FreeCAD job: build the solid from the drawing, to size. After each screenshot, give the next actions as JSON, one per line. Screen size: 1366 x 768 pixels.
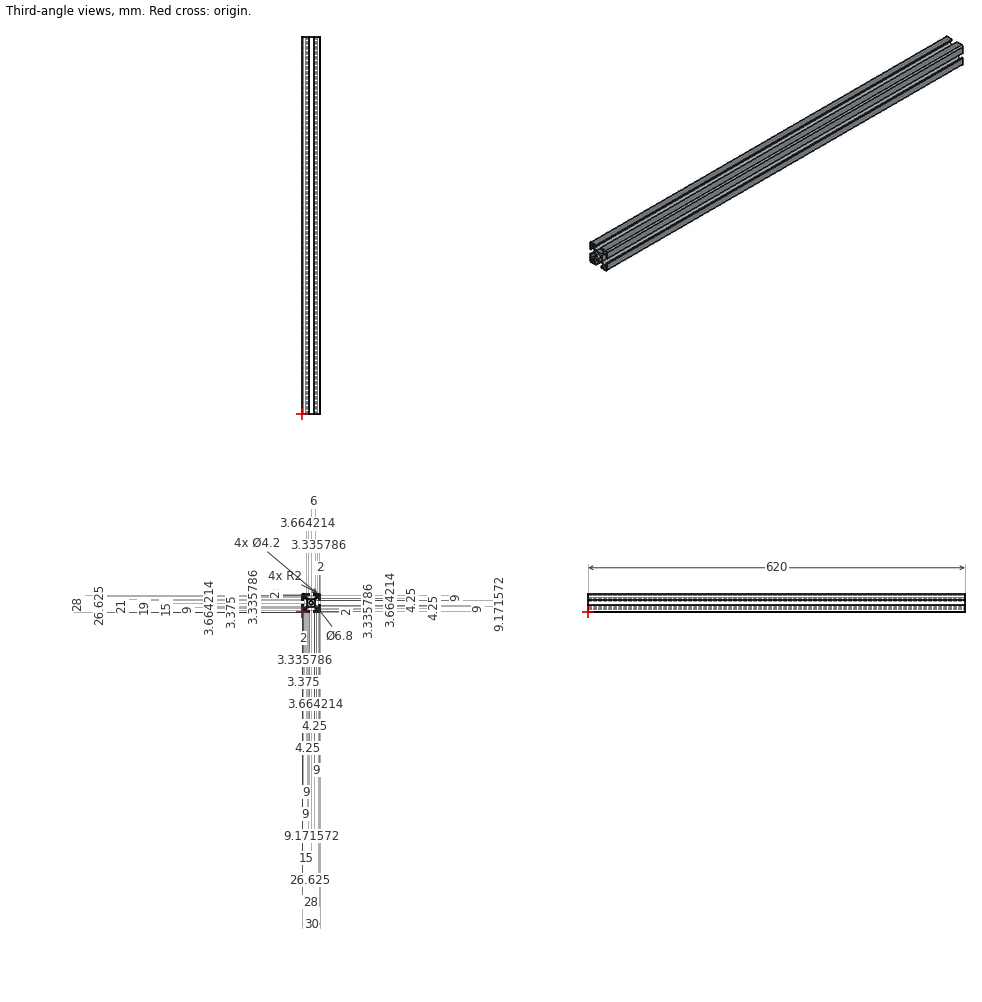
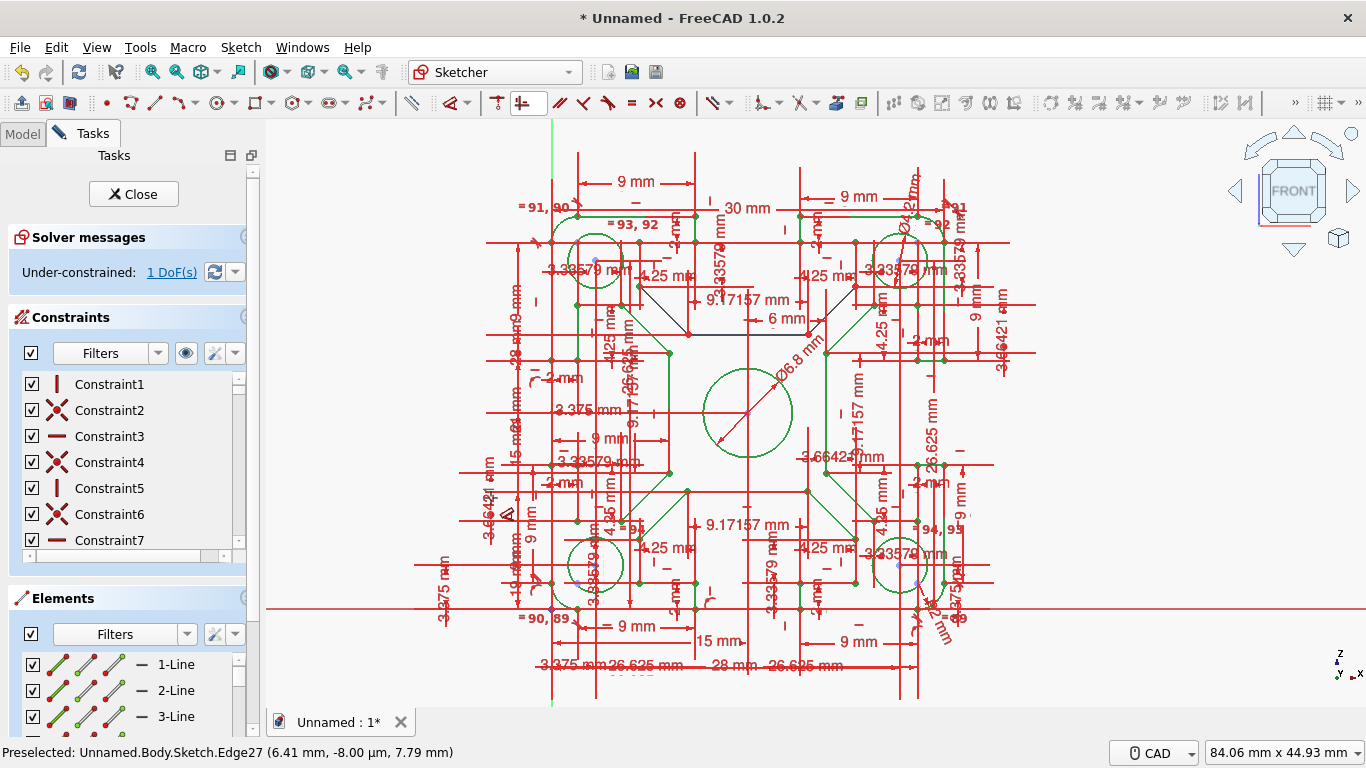
{"action": "left_click", "coordinate": [654, 301]}
{"action": "left_click", "coordinate": [664, 157]}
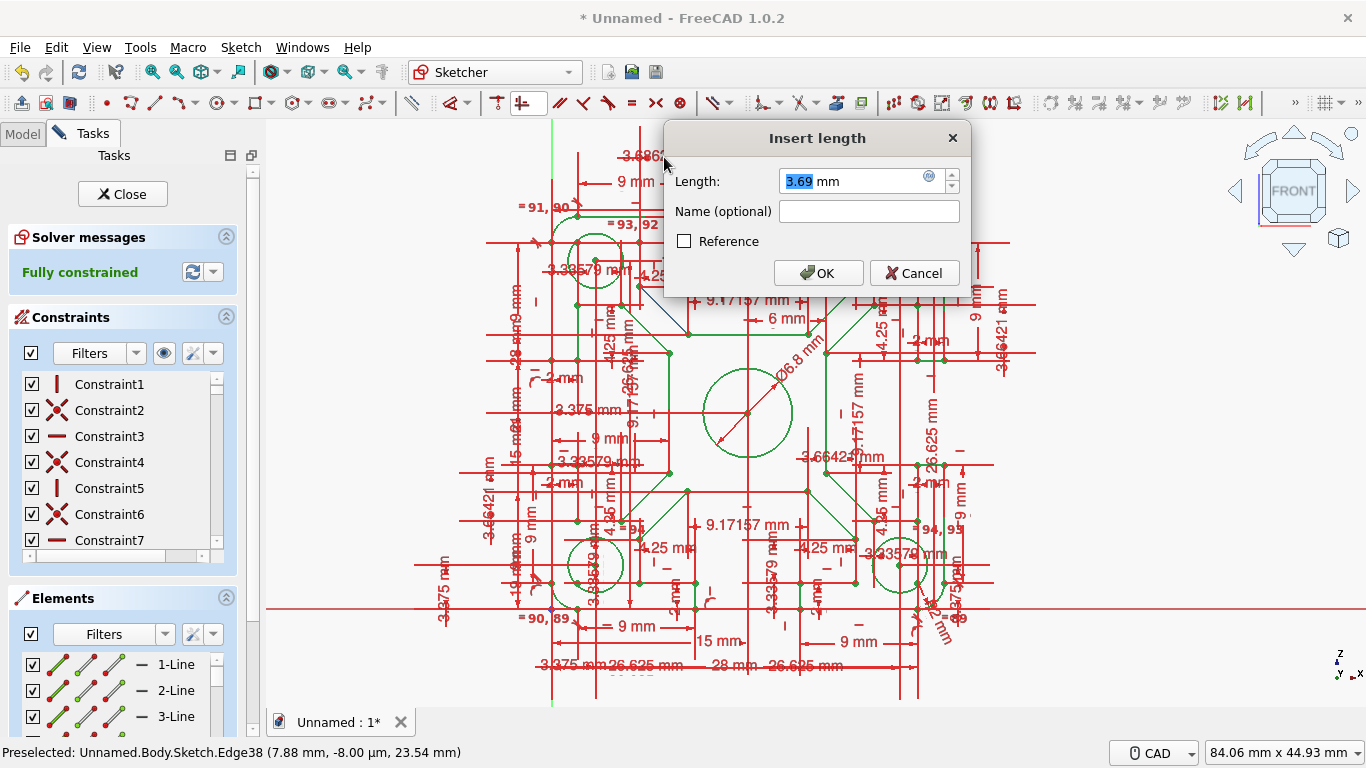
{"action": "type", "text": "3.664214"}
{"action": "key", "text": "Return"}
{"action": "key", "text": "Escape"}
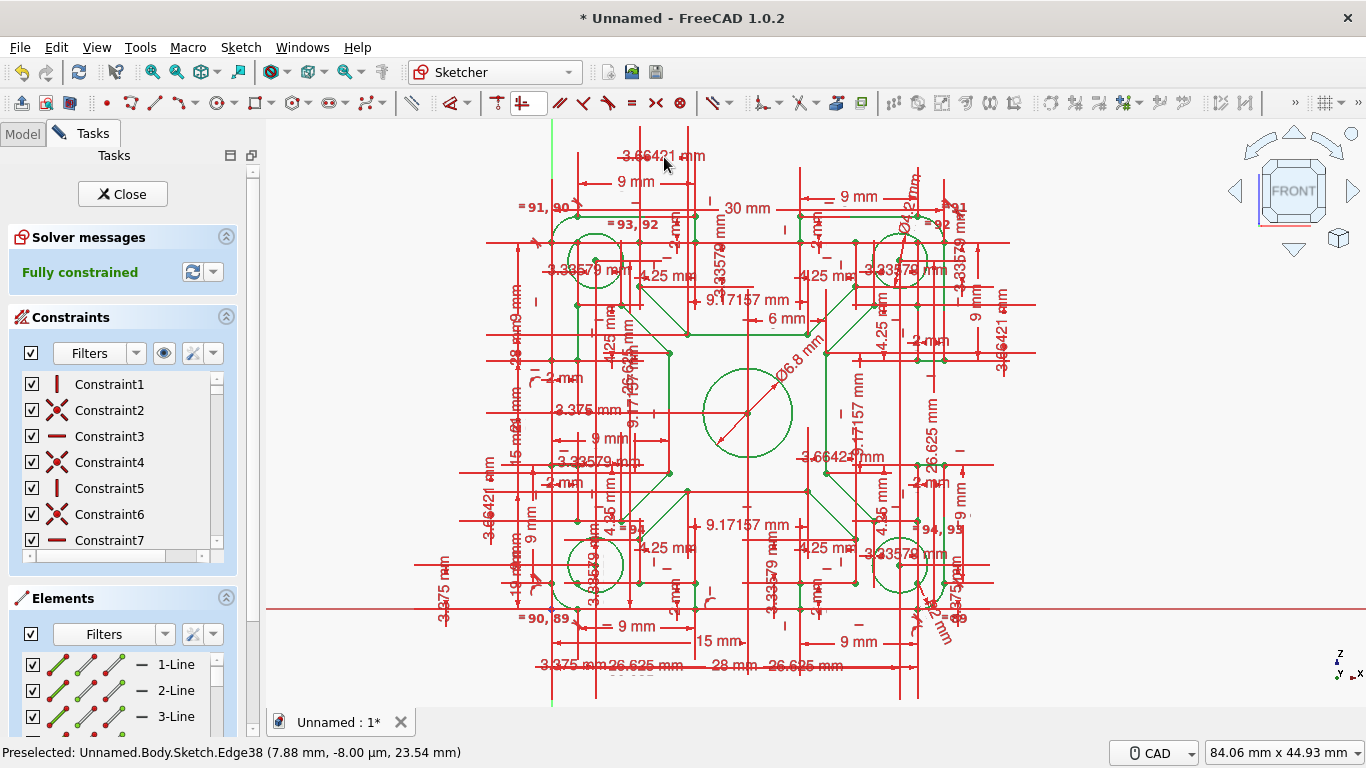
{"action": "left_click", "coordinate": [123, 194]}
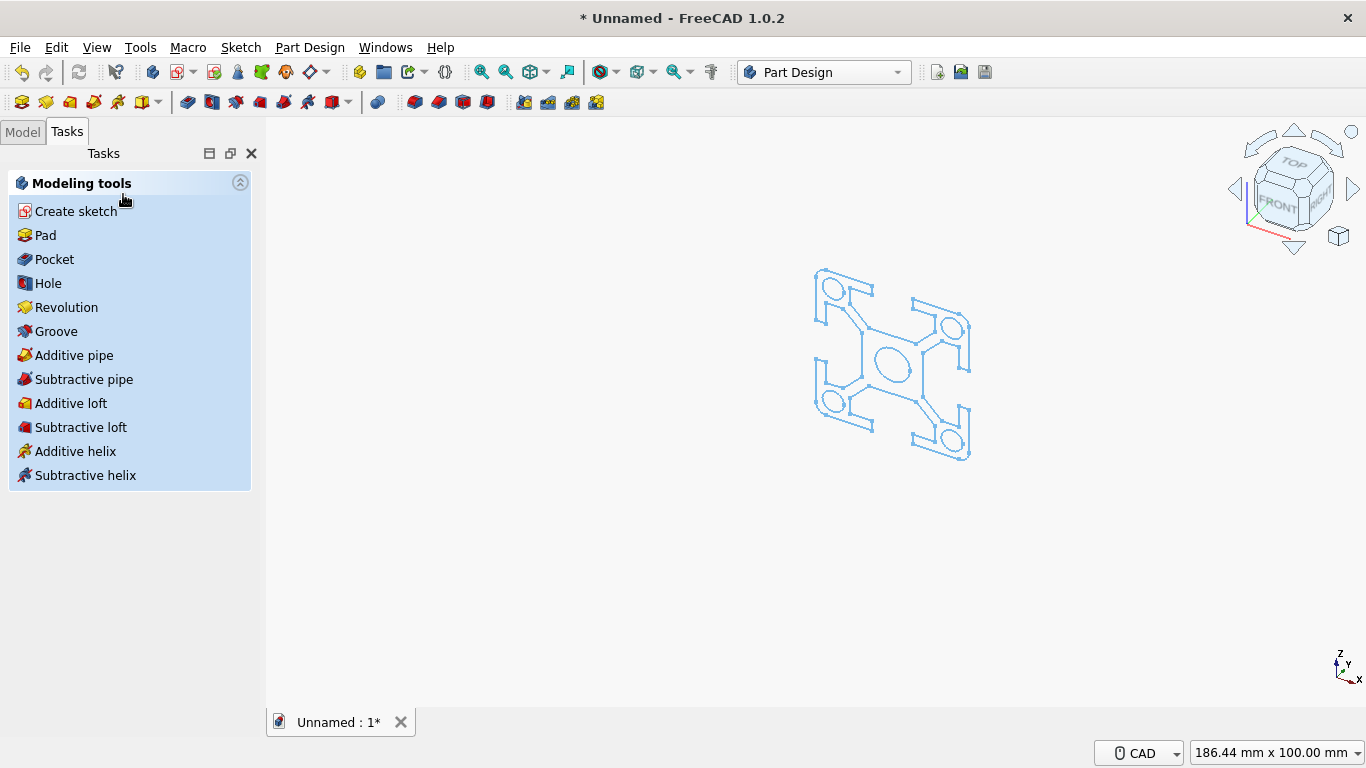
{"action": "left_click", "coordinate": [22, 102]}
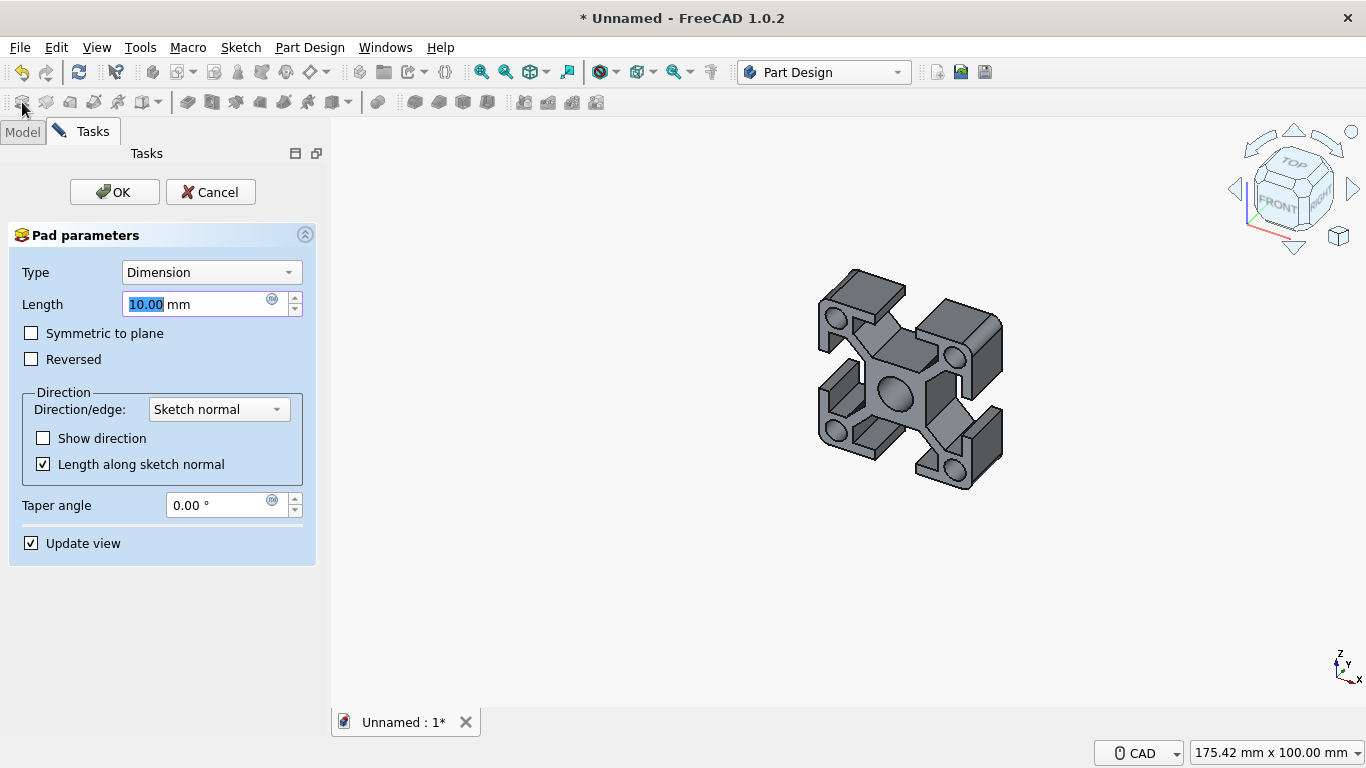
{"action": "type", "text": "620"}
{"action": "key", "text": "Tab"}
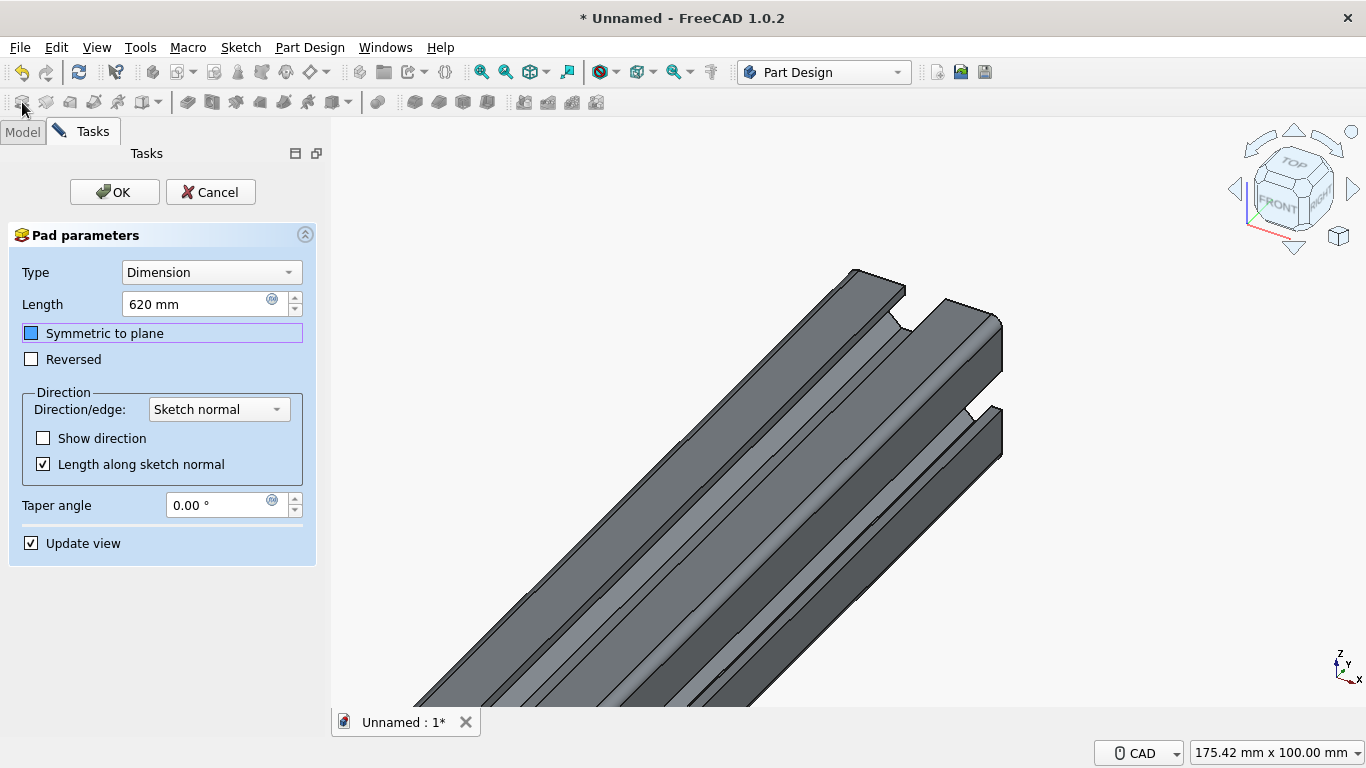
{"action": "left_click", "coordinate": [30, 359]}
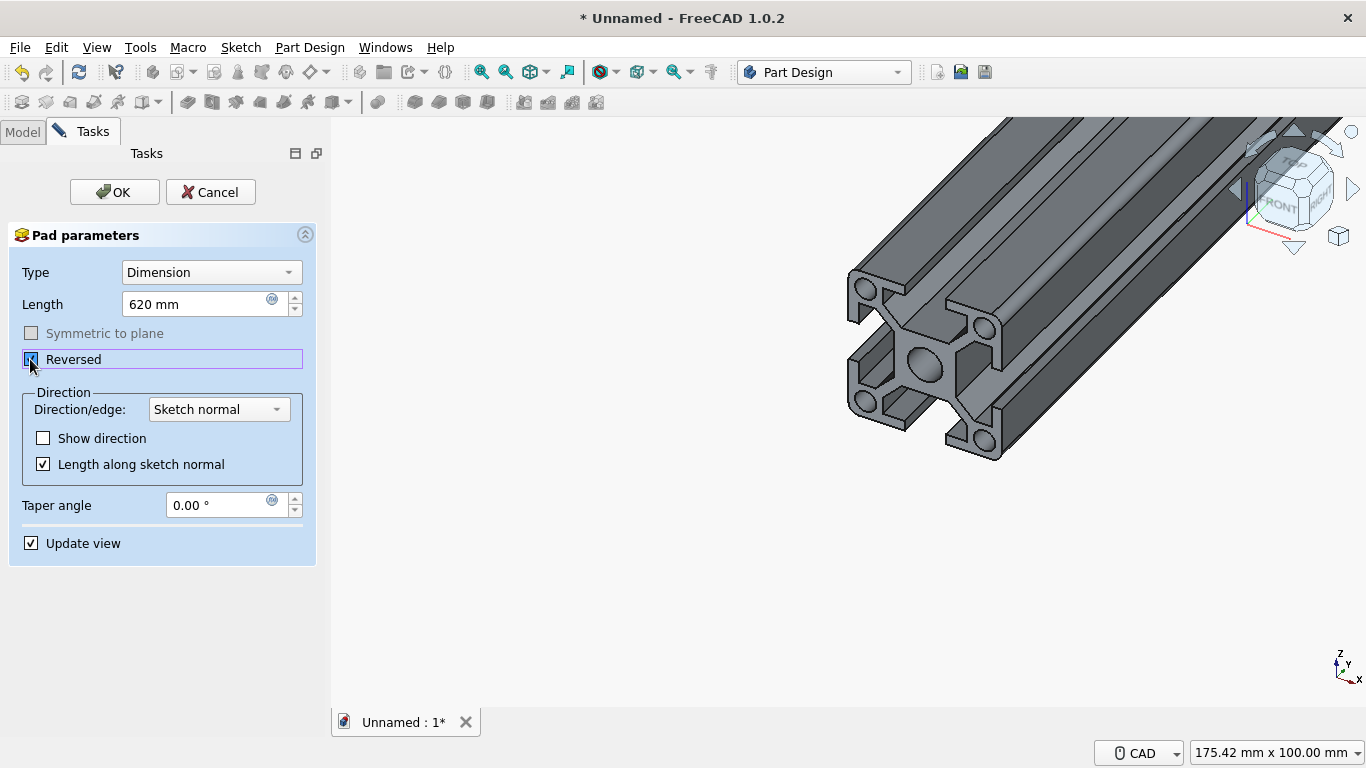
{"action": "left_click", "coordinate": [115, 192]}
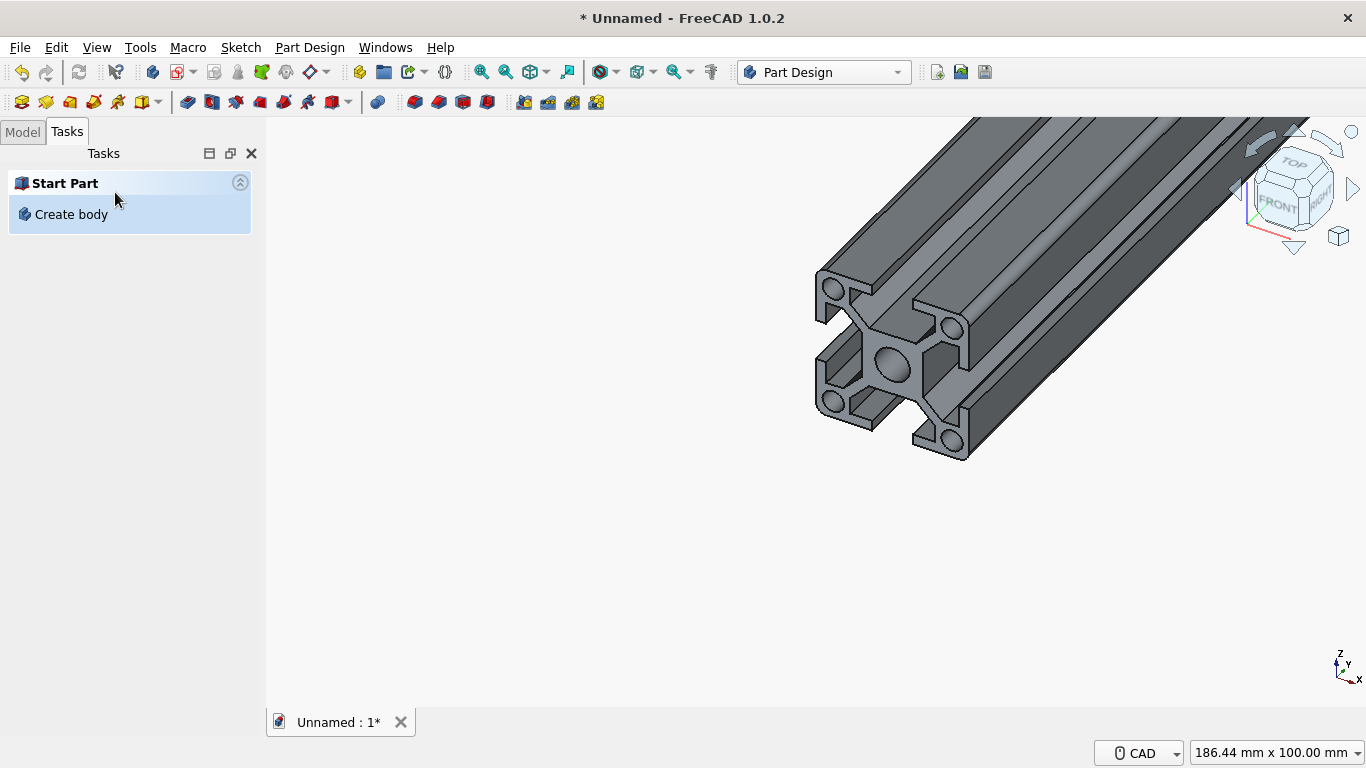
{"action": "key", "text": "0"}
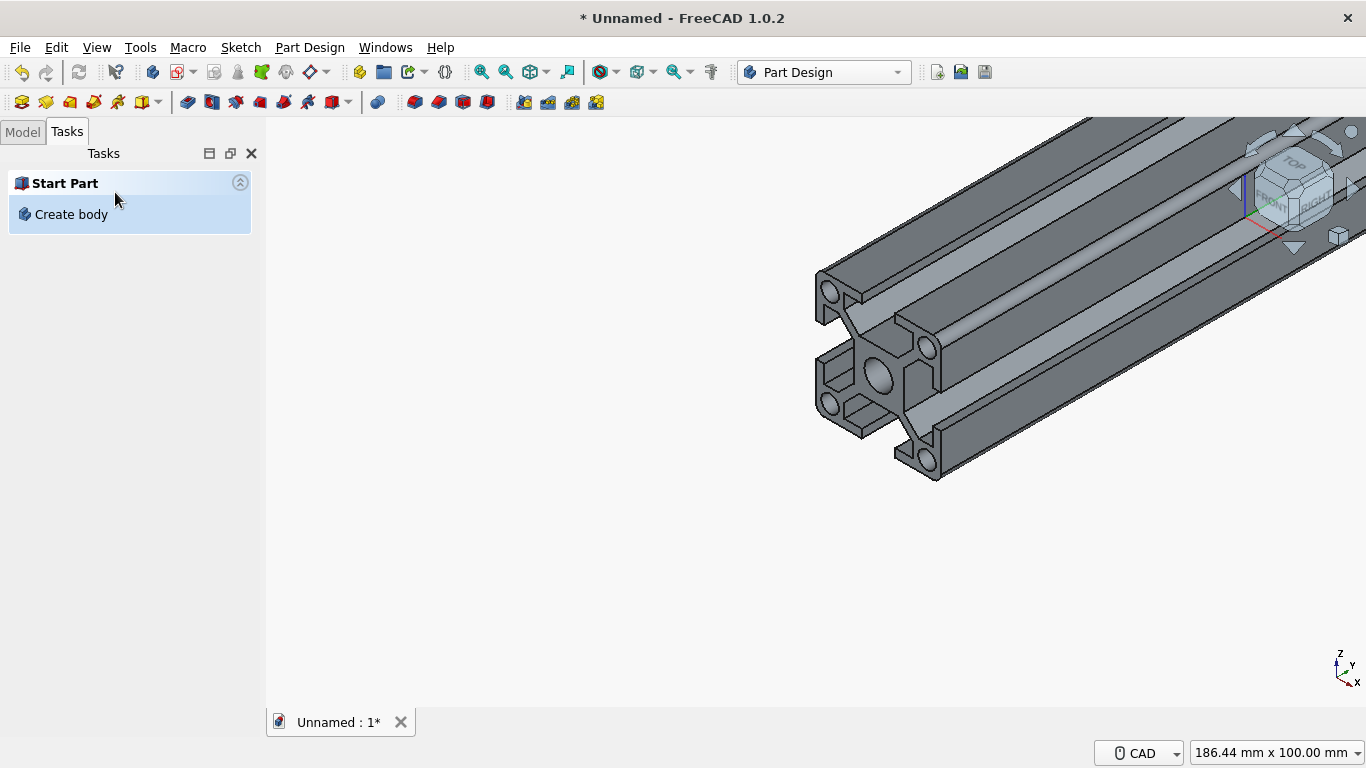
{"action": "left_click", "coordinate": [482, 72]}